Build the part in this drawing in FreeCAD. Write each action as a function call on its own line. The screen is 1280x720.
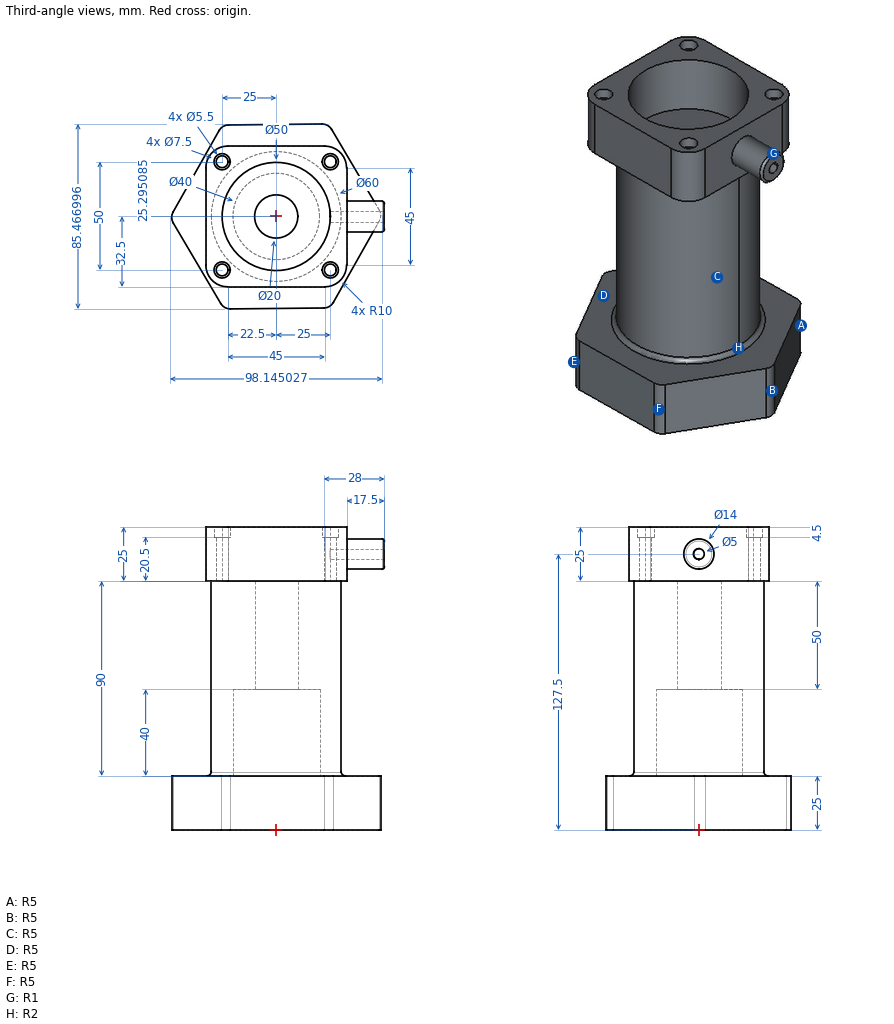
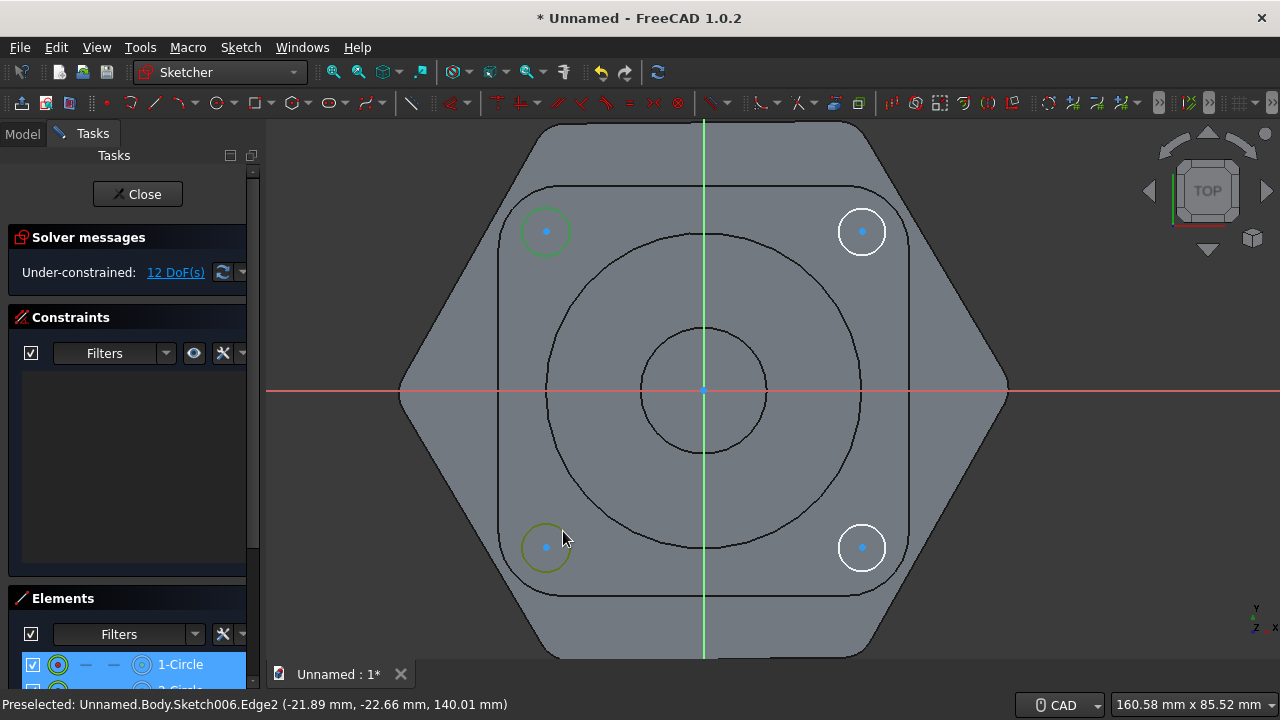
click(878, 531)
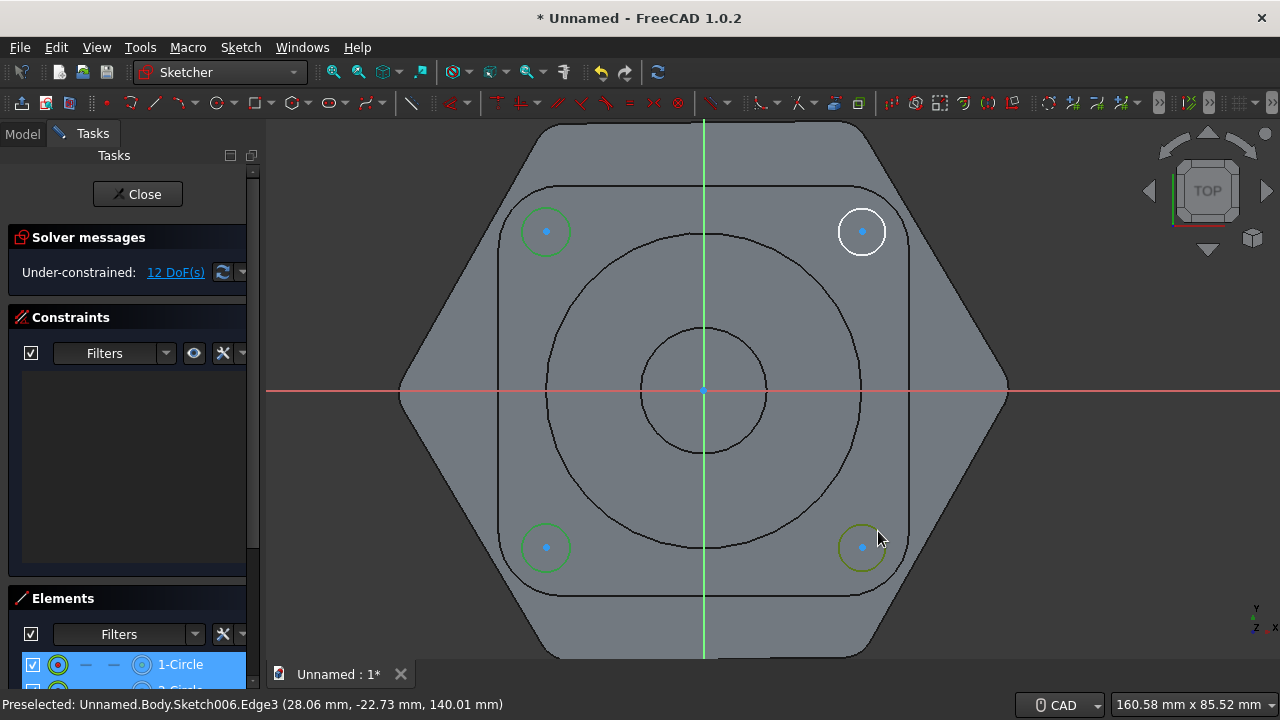
click(878, 215)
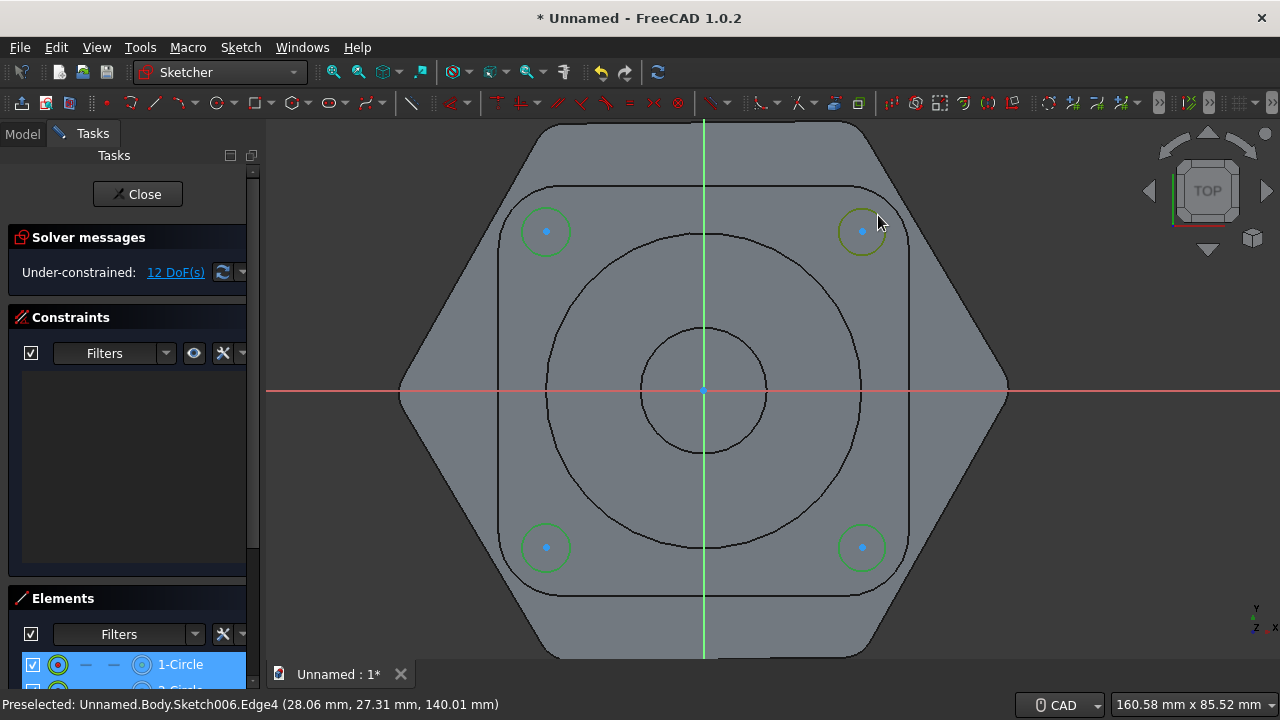
click(630, 104)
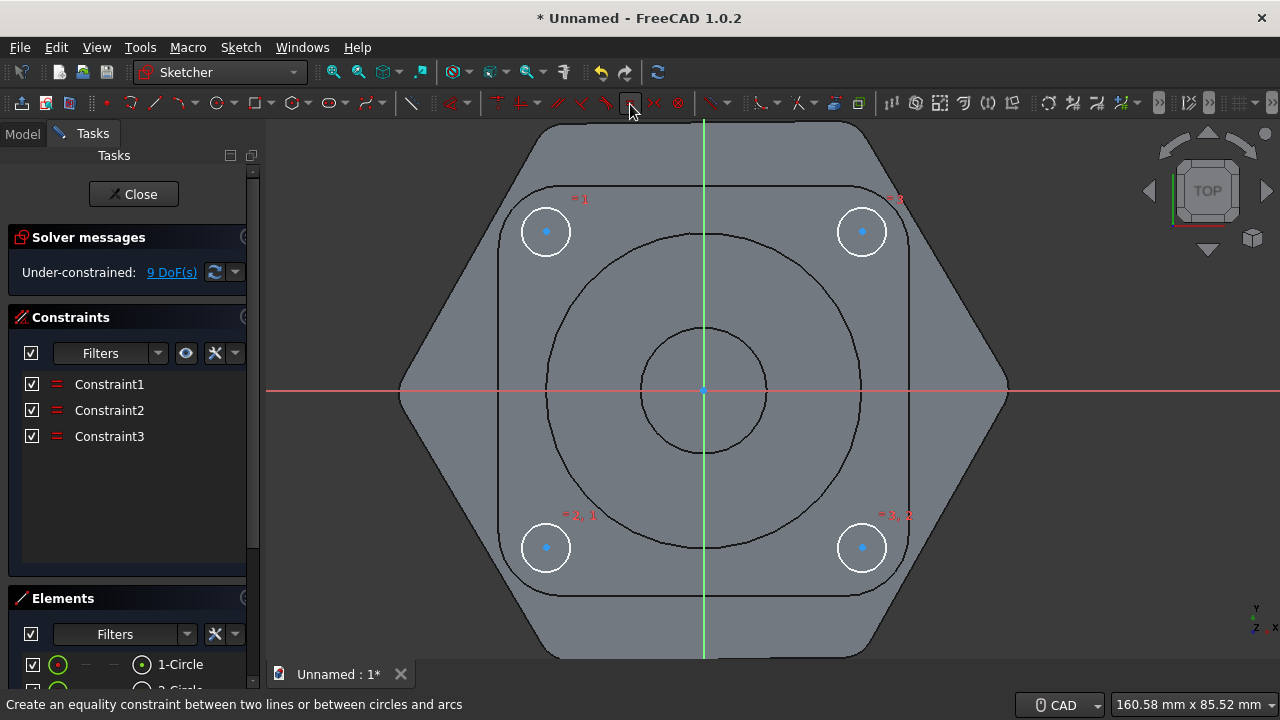
click(546, 232)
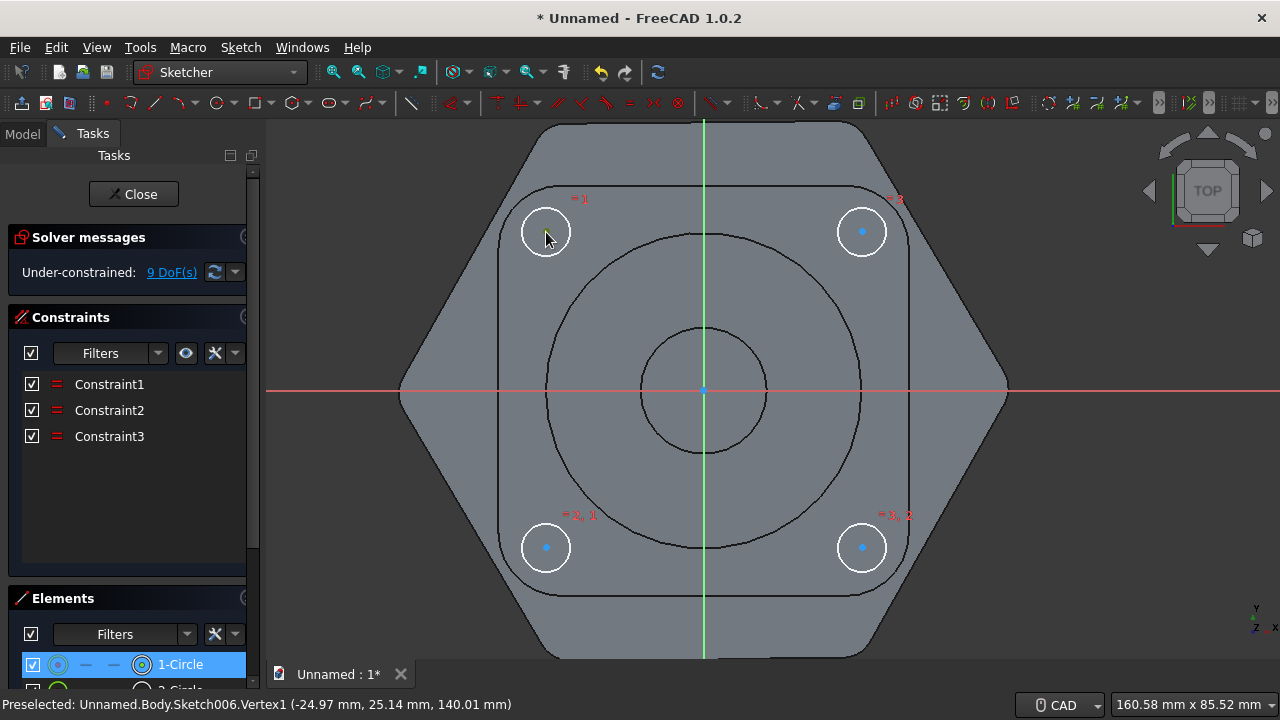
click(546, 548)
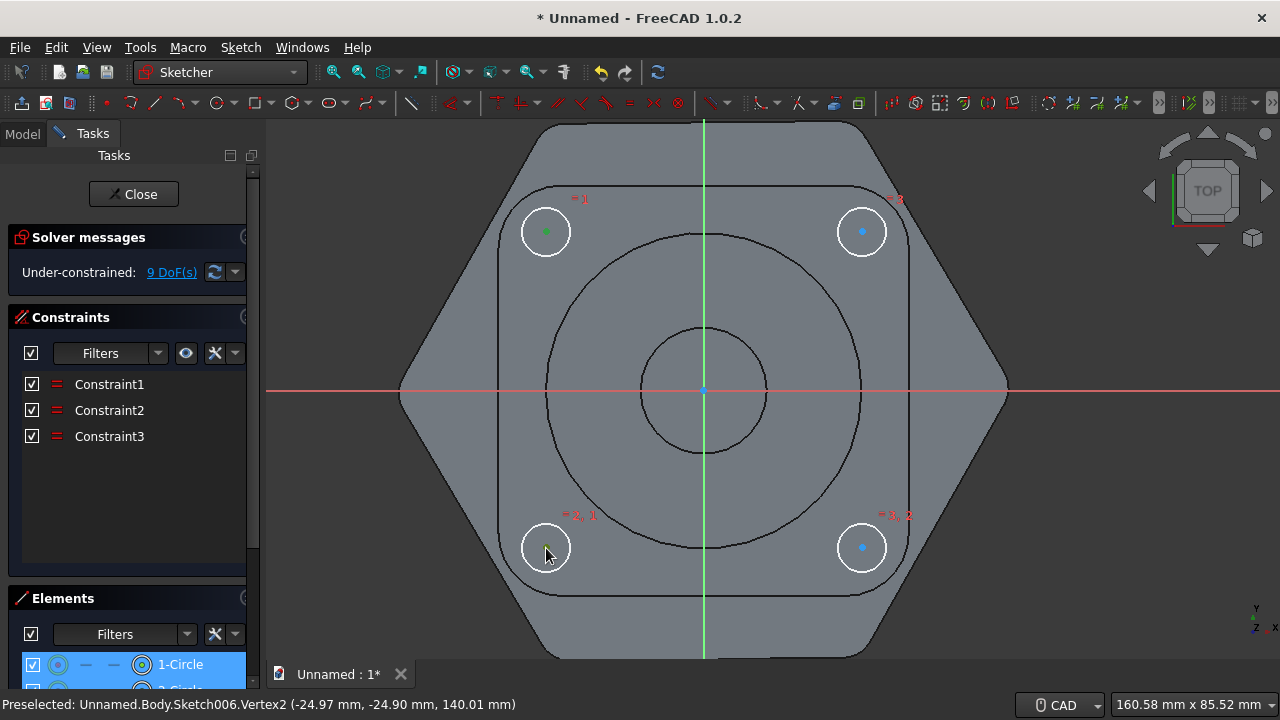
key(v)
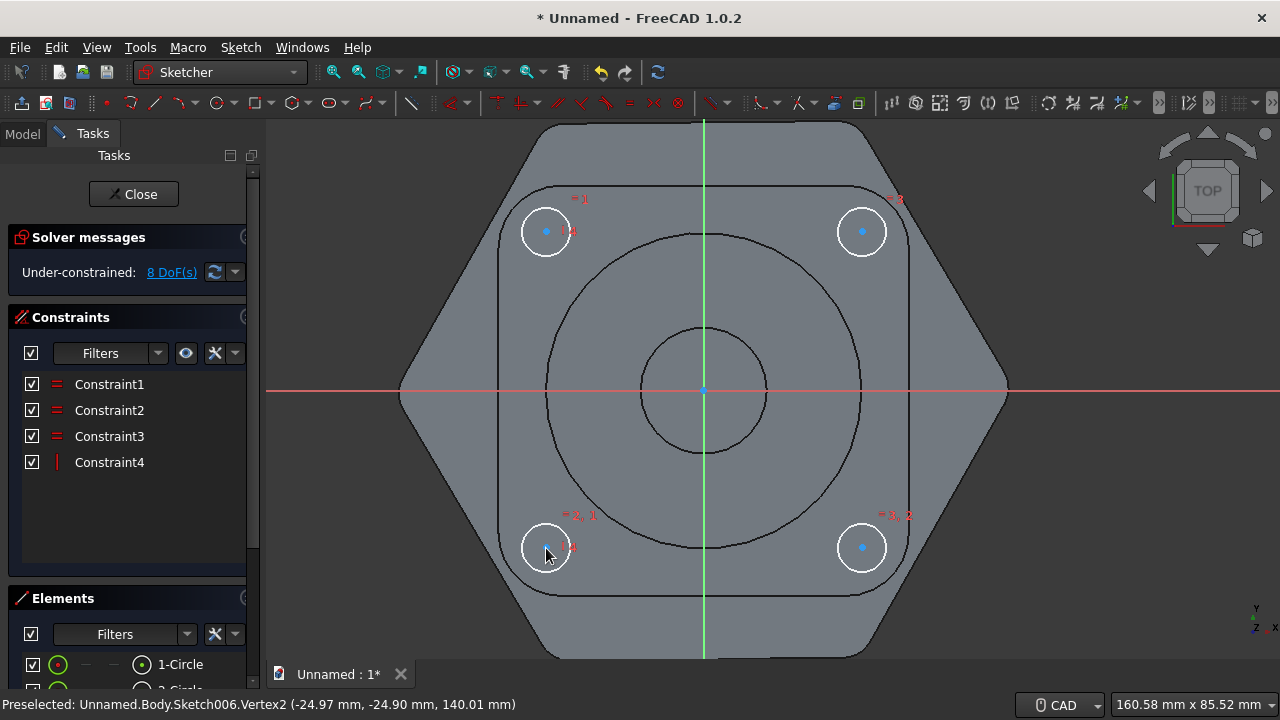
click(546, 548)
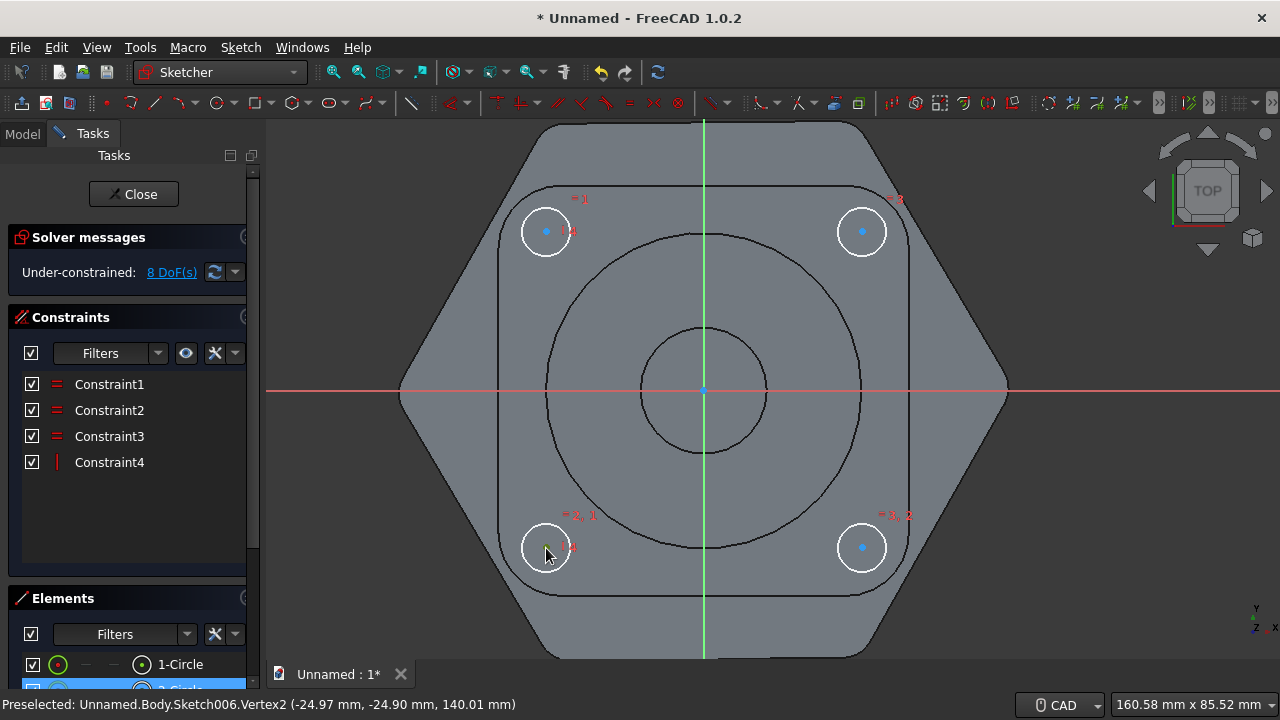
click(862, 548)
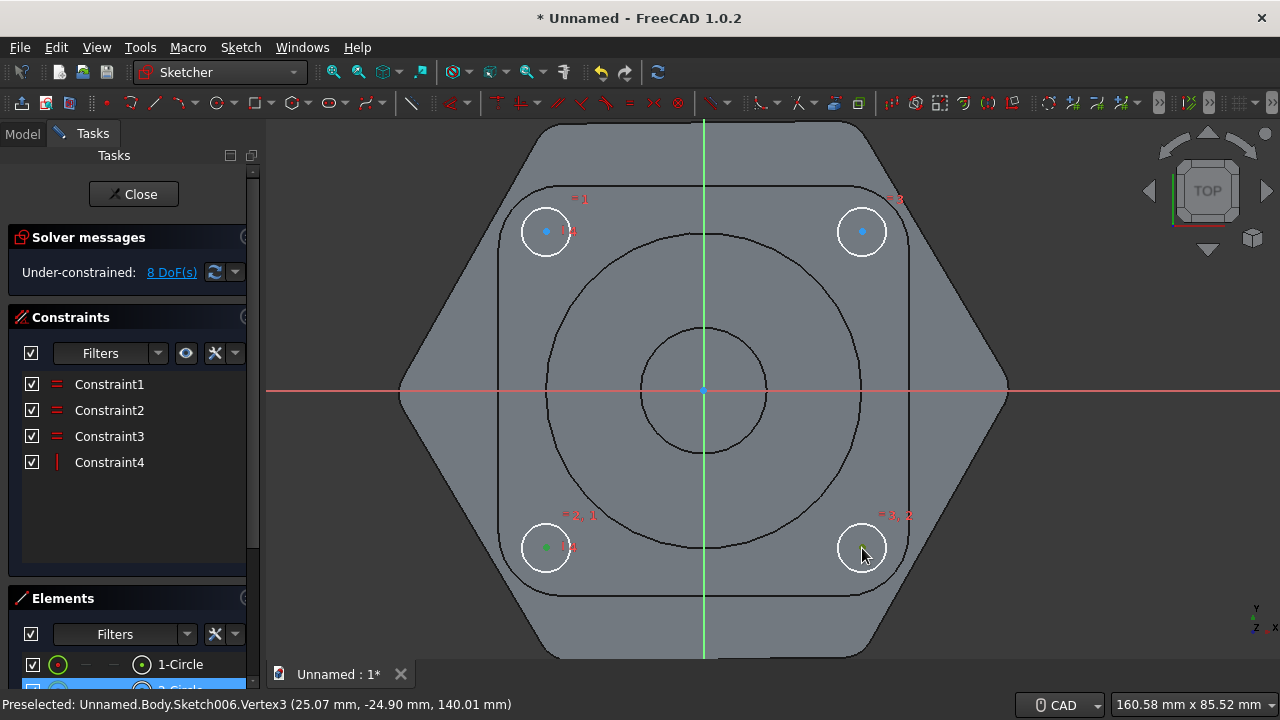
click(540, 104)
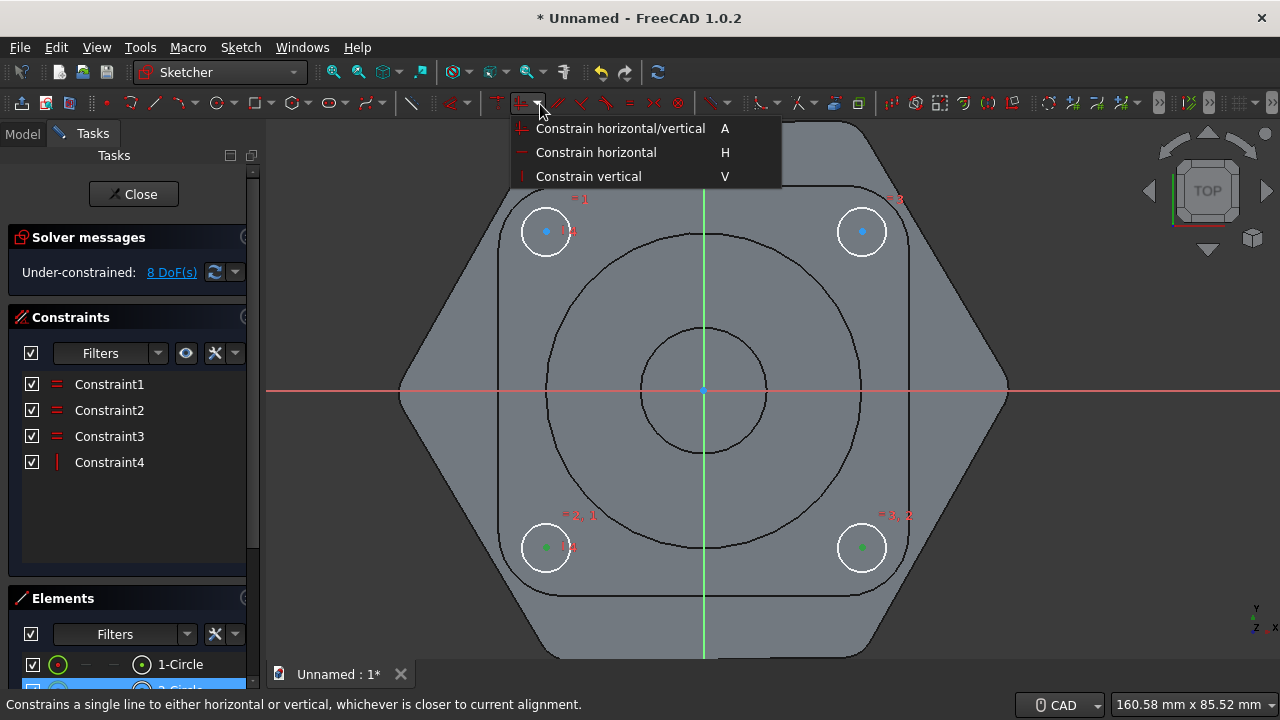
click(646, 152)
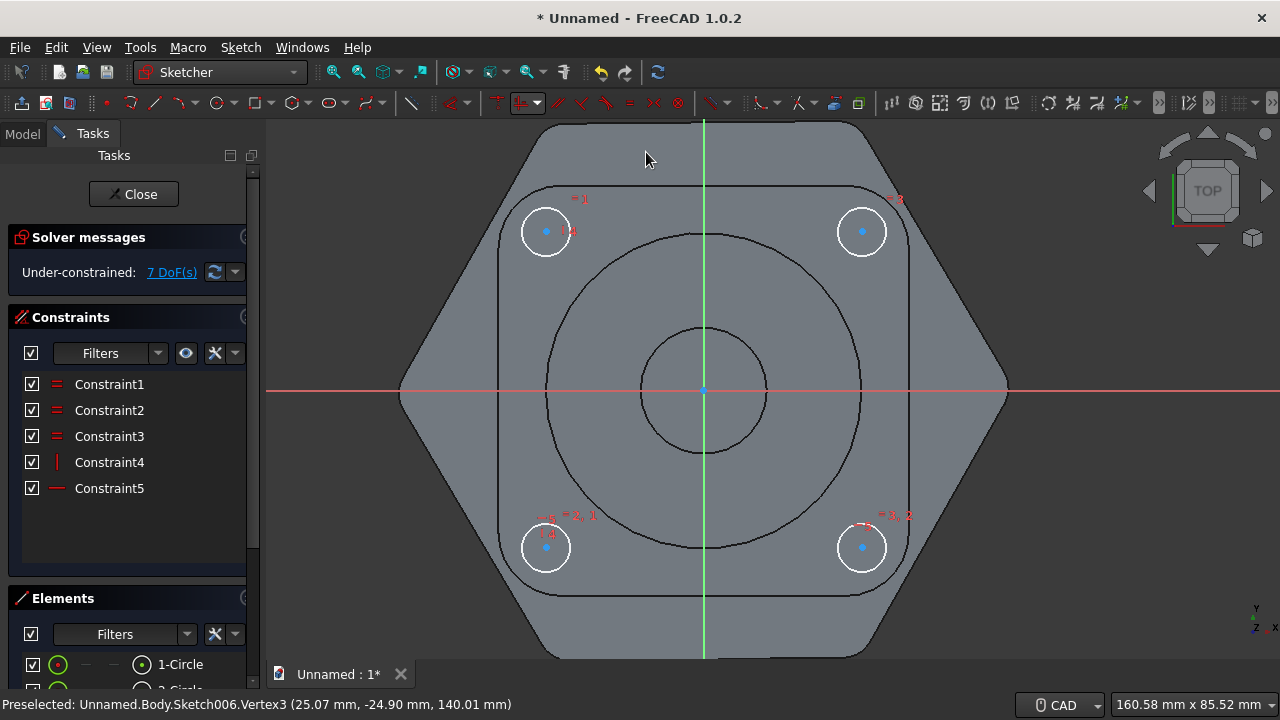
click(862, 548)